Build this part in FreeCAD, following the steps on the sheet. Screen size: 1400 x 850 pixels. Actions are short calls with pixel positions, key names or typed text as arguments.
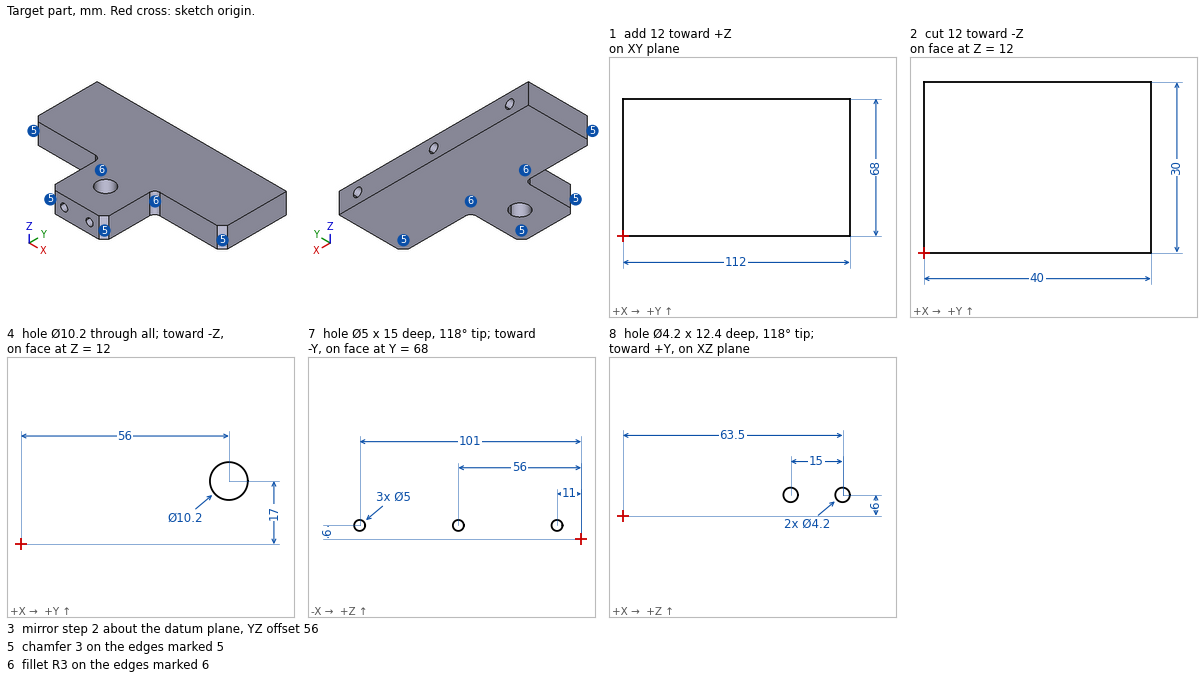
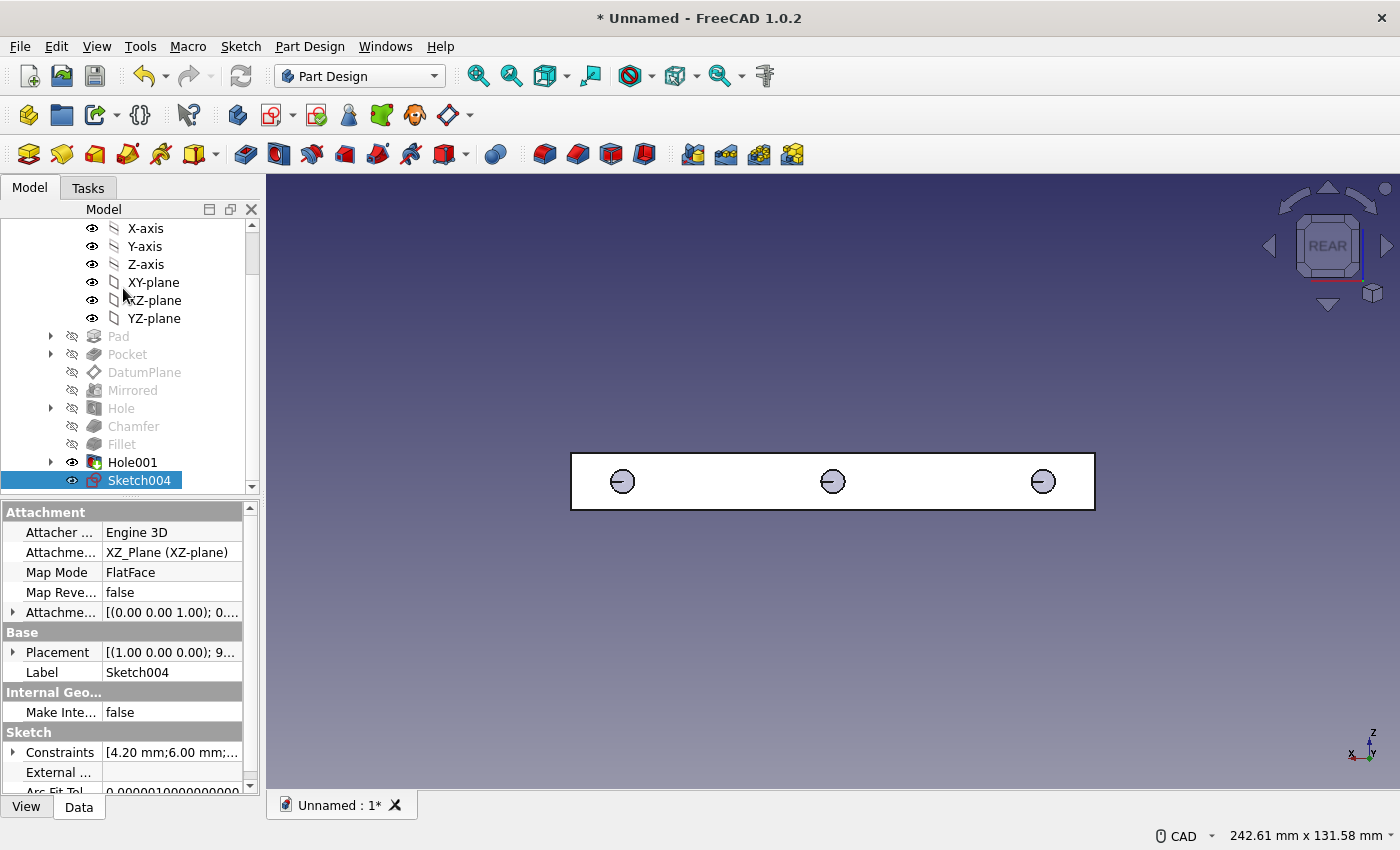
click(279, 154)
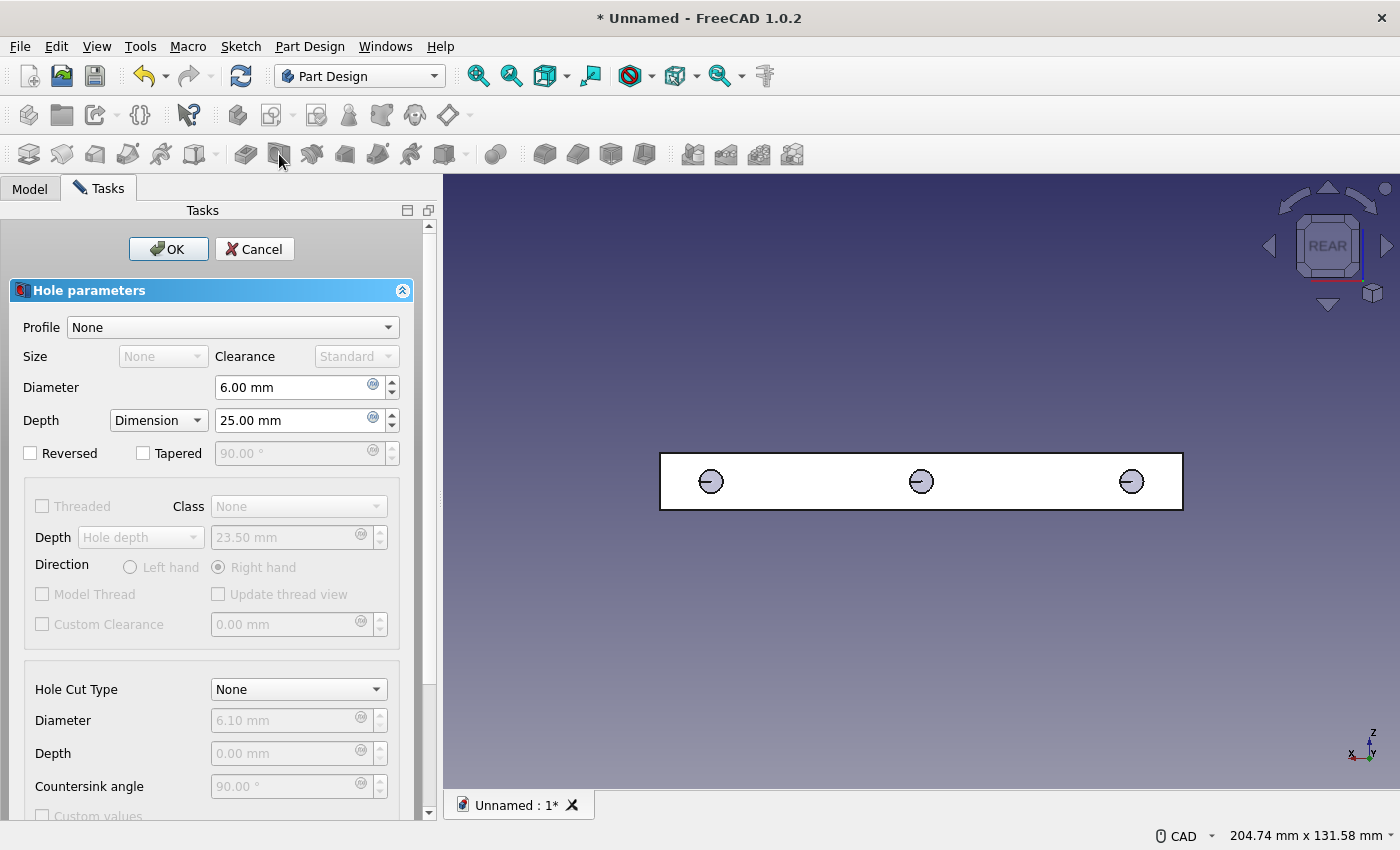
triple_click(300, 388)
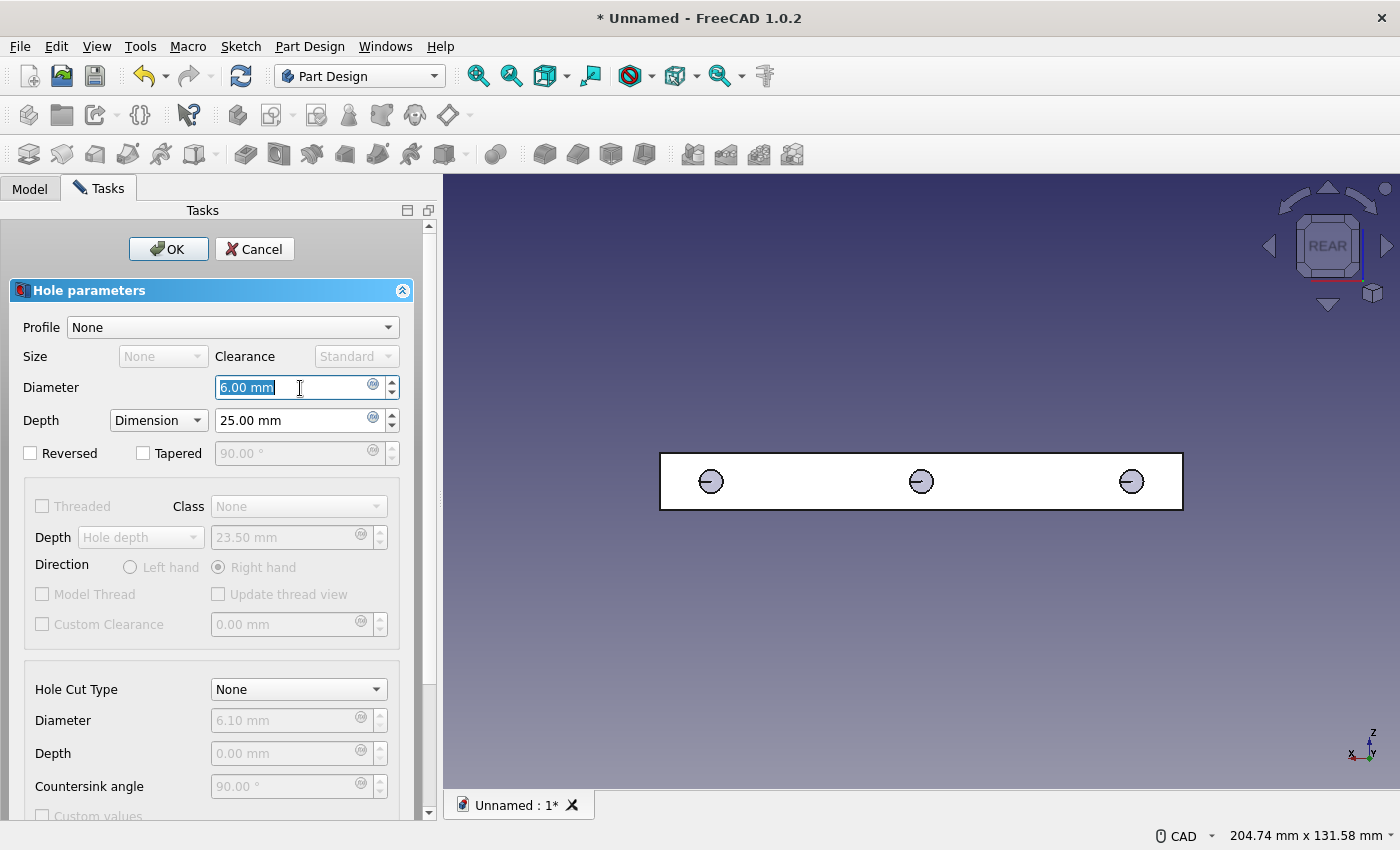
text(4.2)
key(Tab)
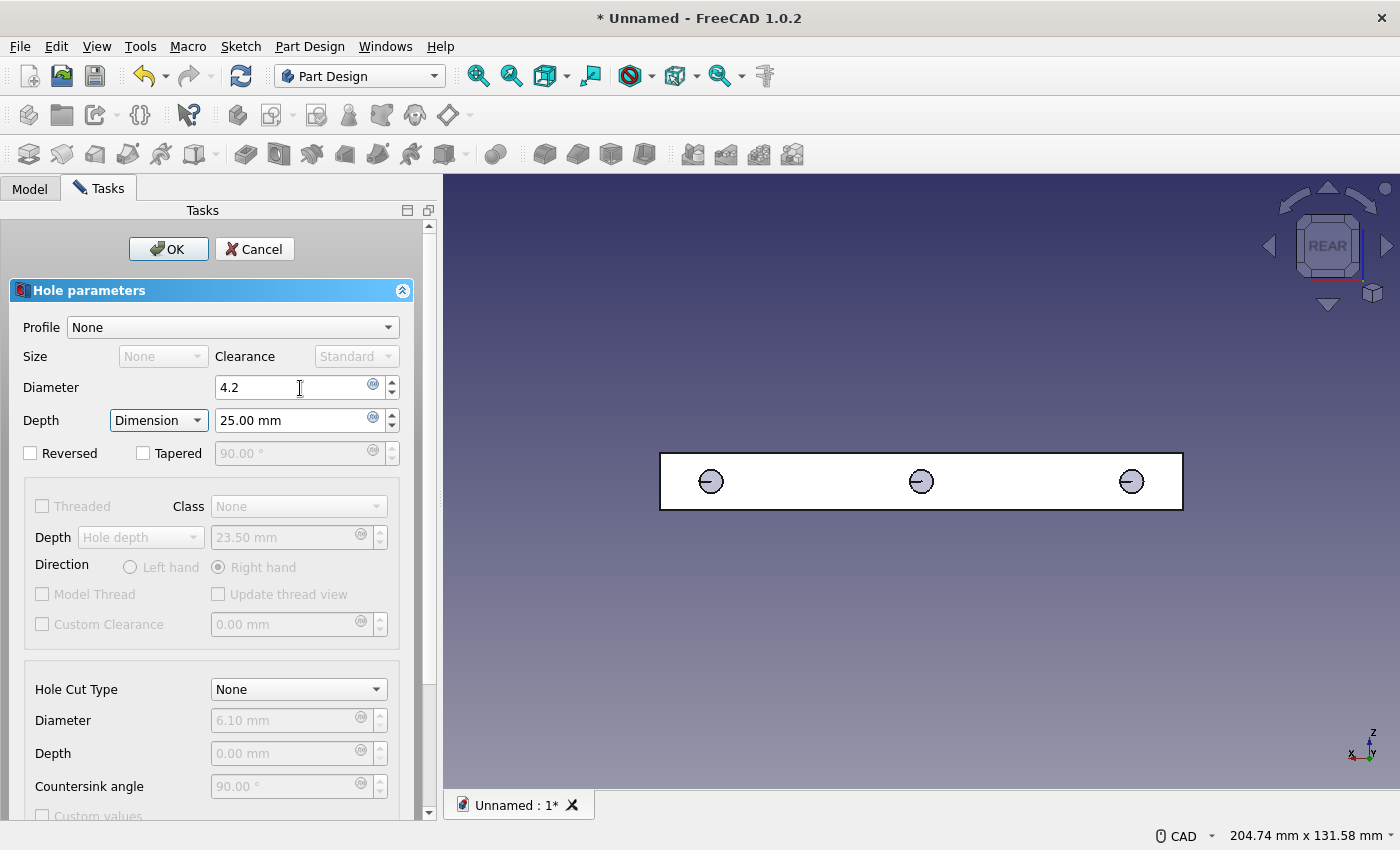
triple_click(300, 420)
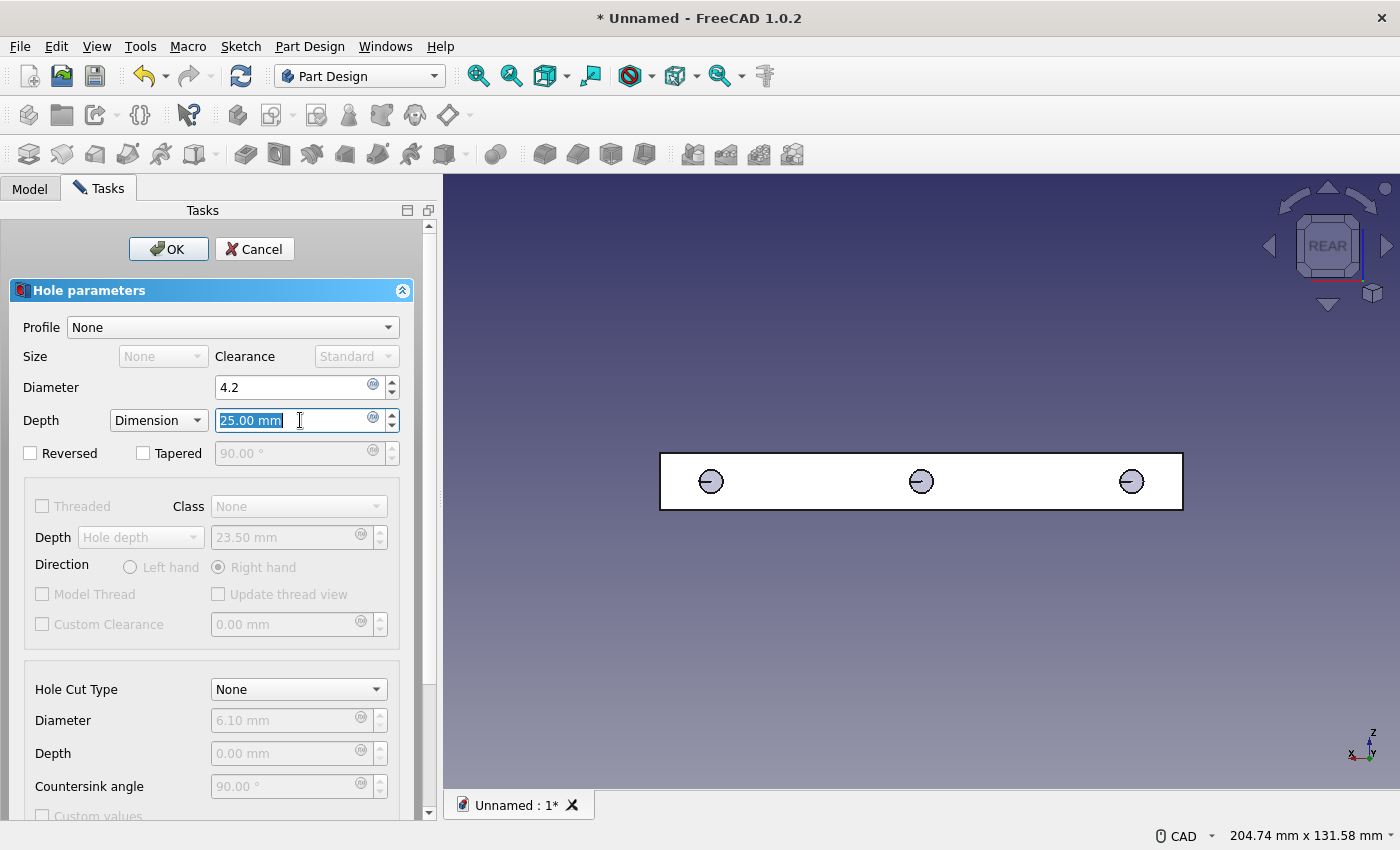
text(12.4)
key(Tab)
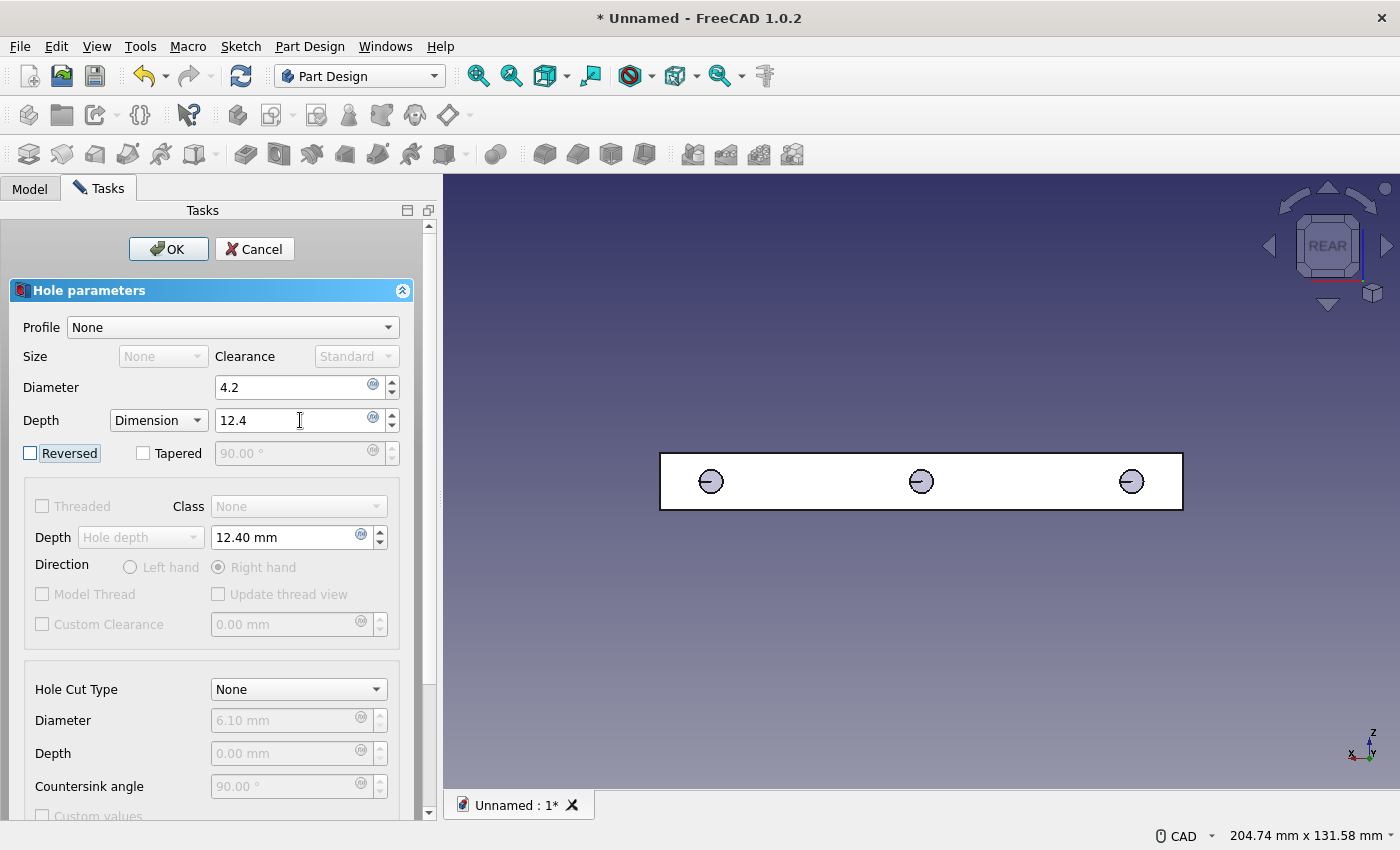
click(169, 249)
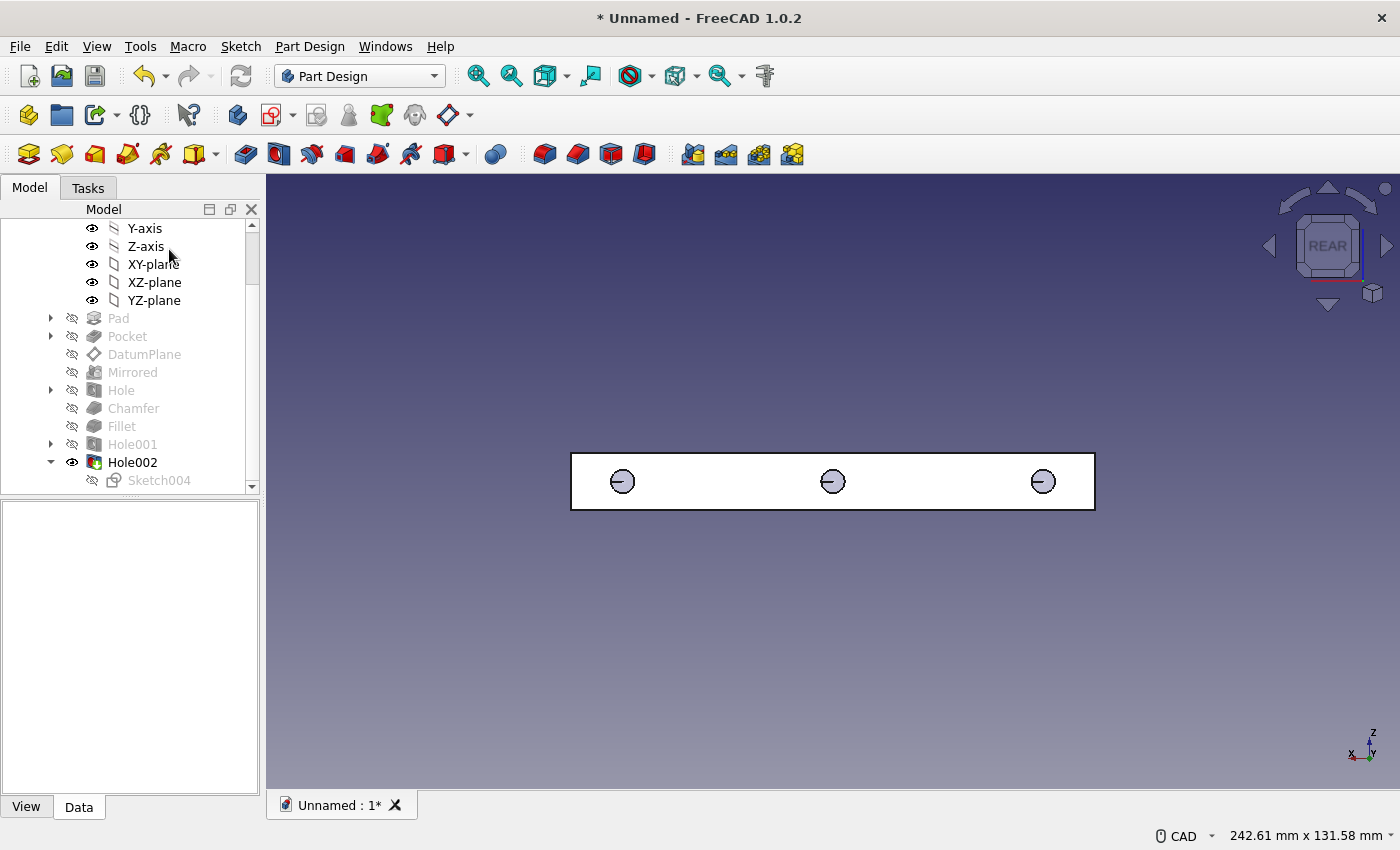
key(0)